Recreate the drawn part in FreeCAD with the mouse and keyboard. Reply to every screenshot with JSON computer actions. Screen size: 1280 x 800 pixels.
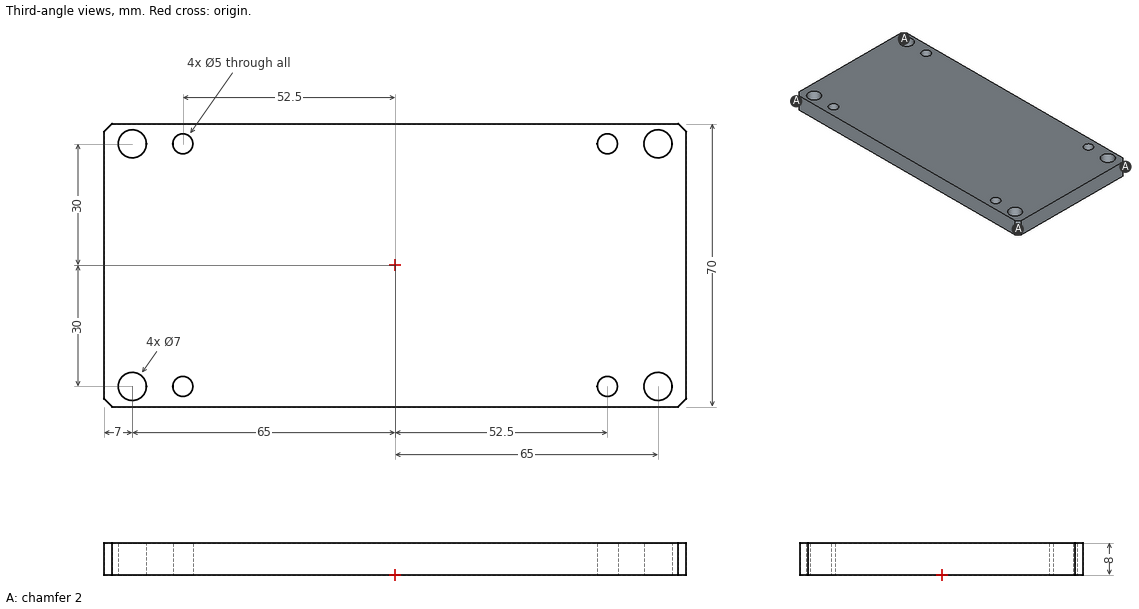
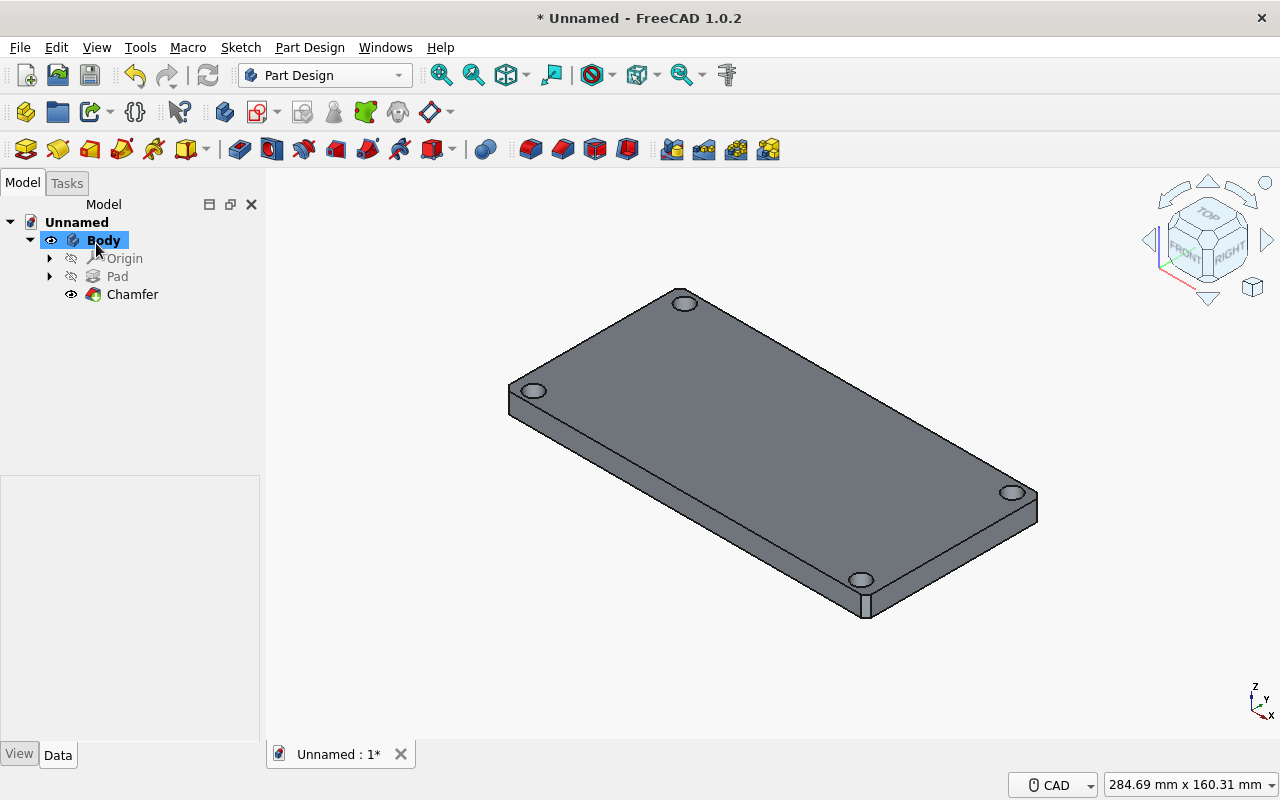
{"action": "left_click", "coordinate": [825, 471]}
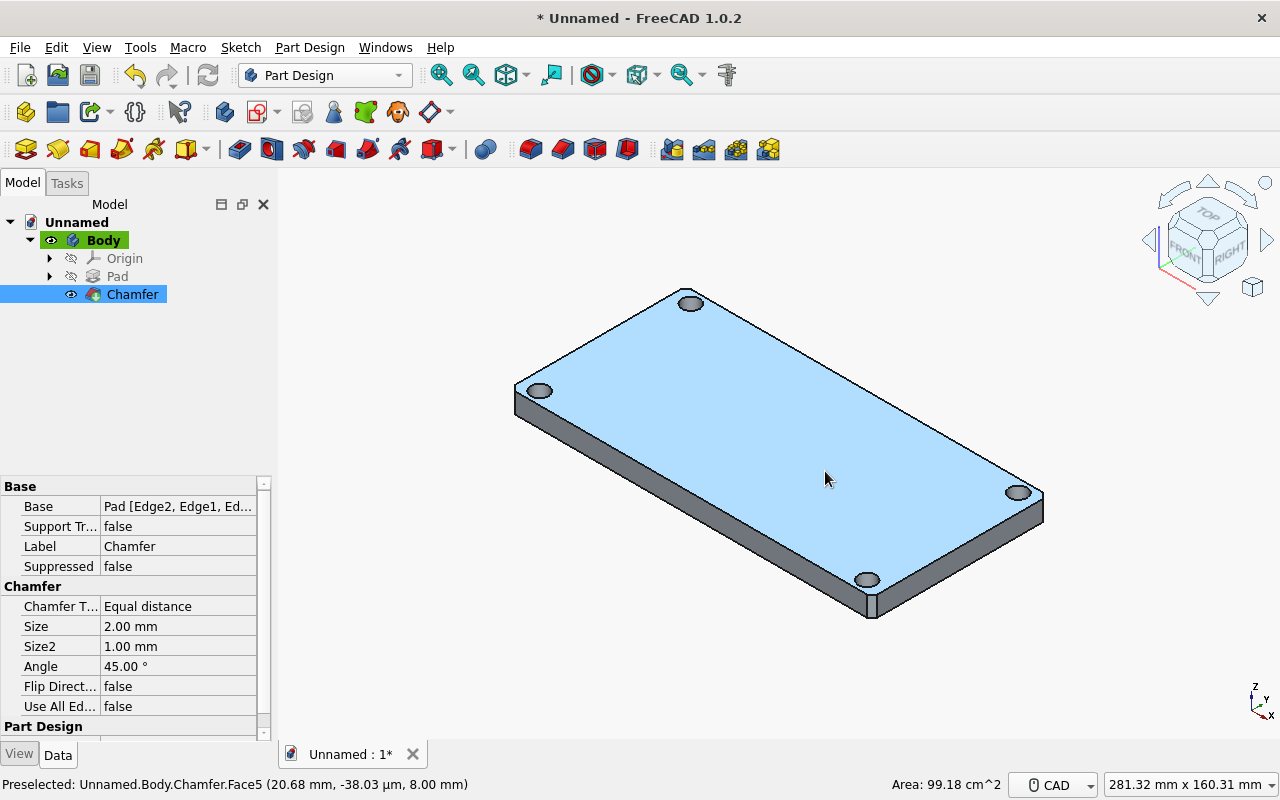
{"action": "left_click", "coordinate": [258, 112]}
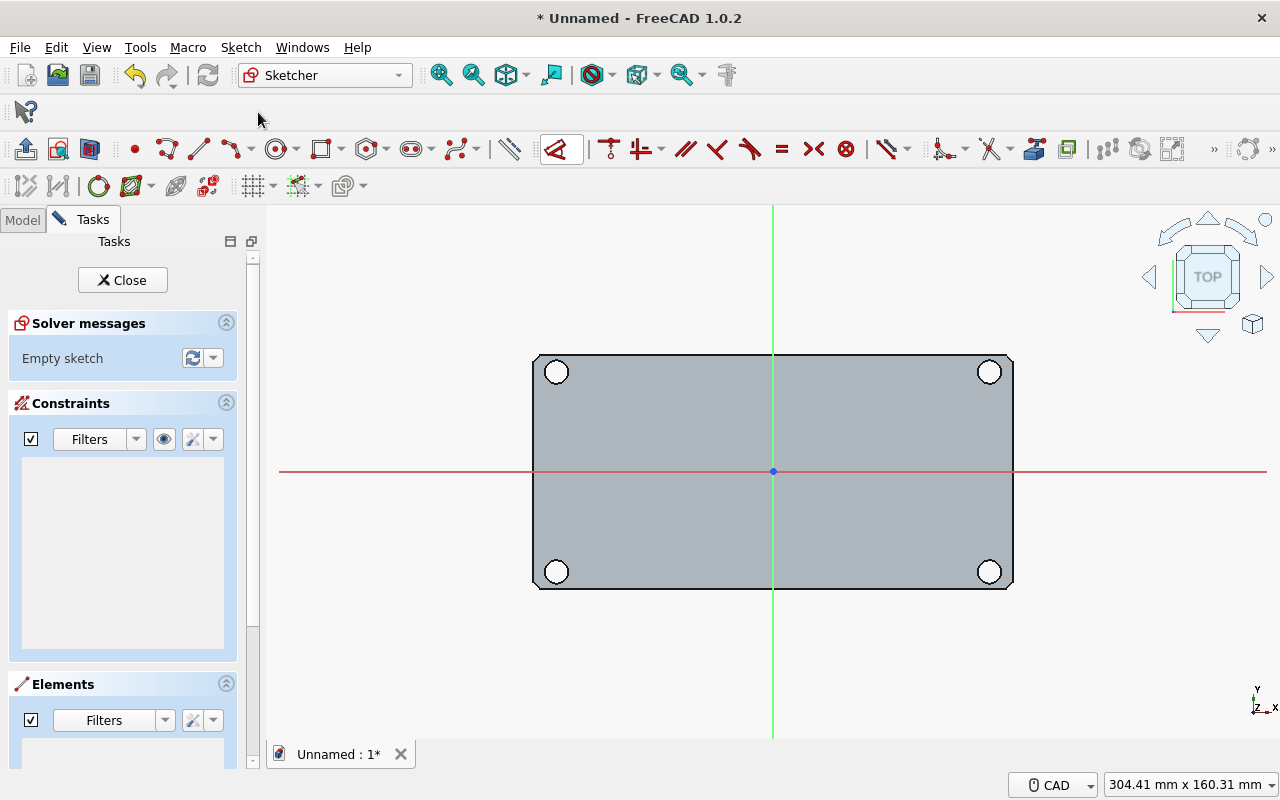
{"action": "scroll", "coordinate": [912, 472], "scroll_direction": "up", "scroll_amount": 2}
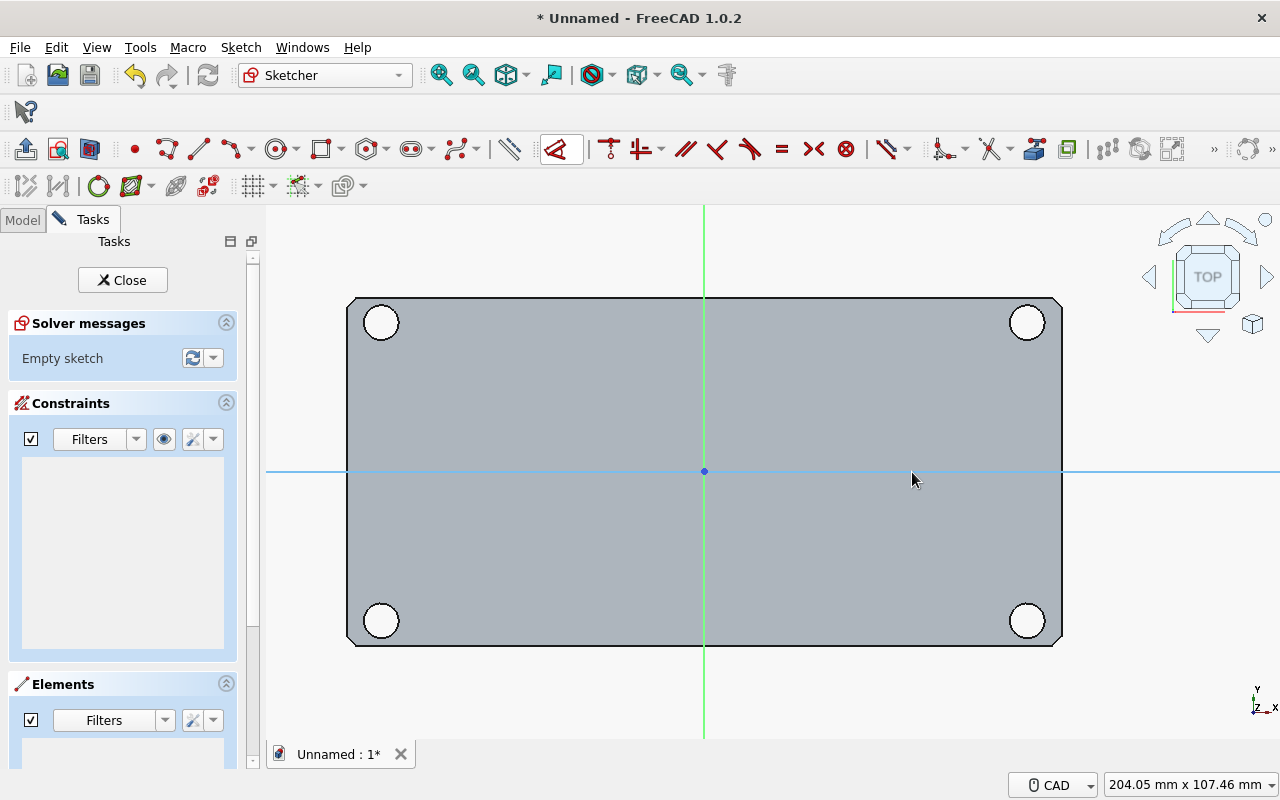
{"action": "left_click", "coordinate": [276, 150]}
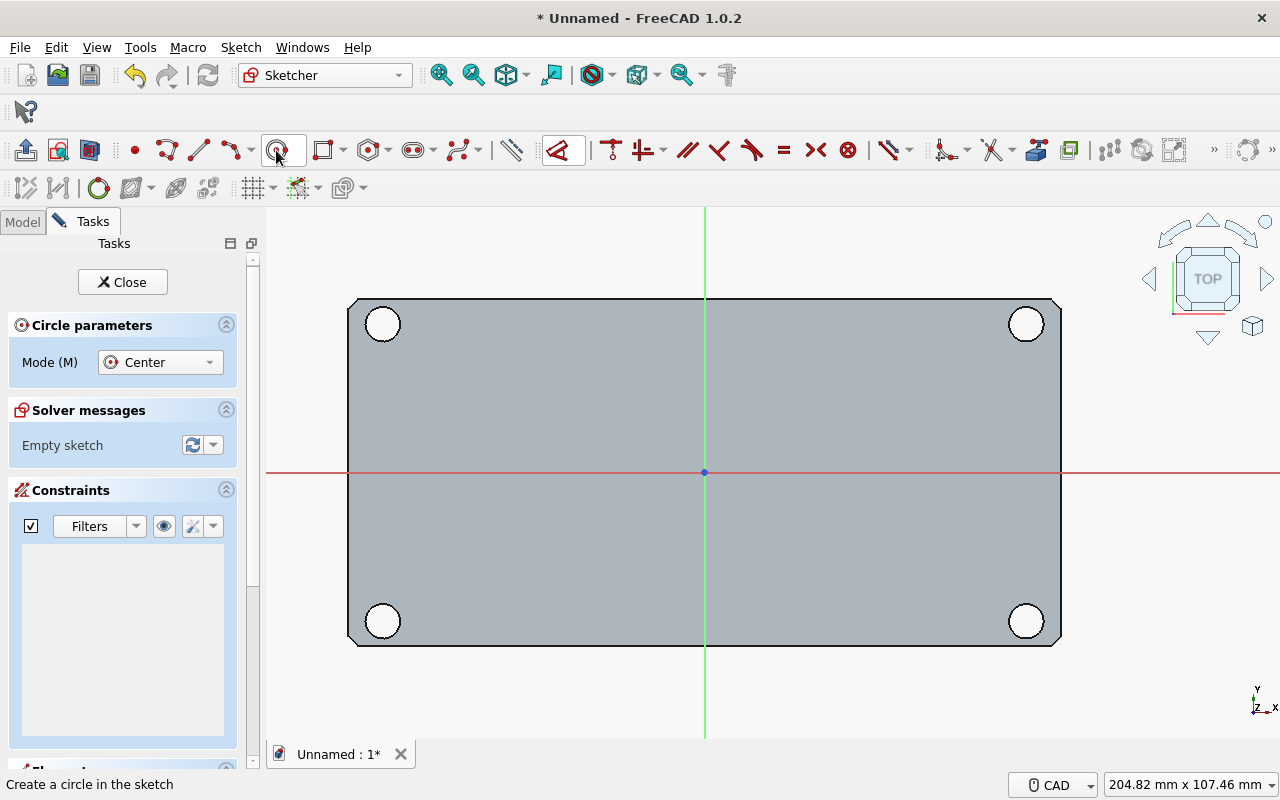
{"action": "scroll", "coordinate": [445, 324], "scroll_direction": "up", "scroll_amount": 4}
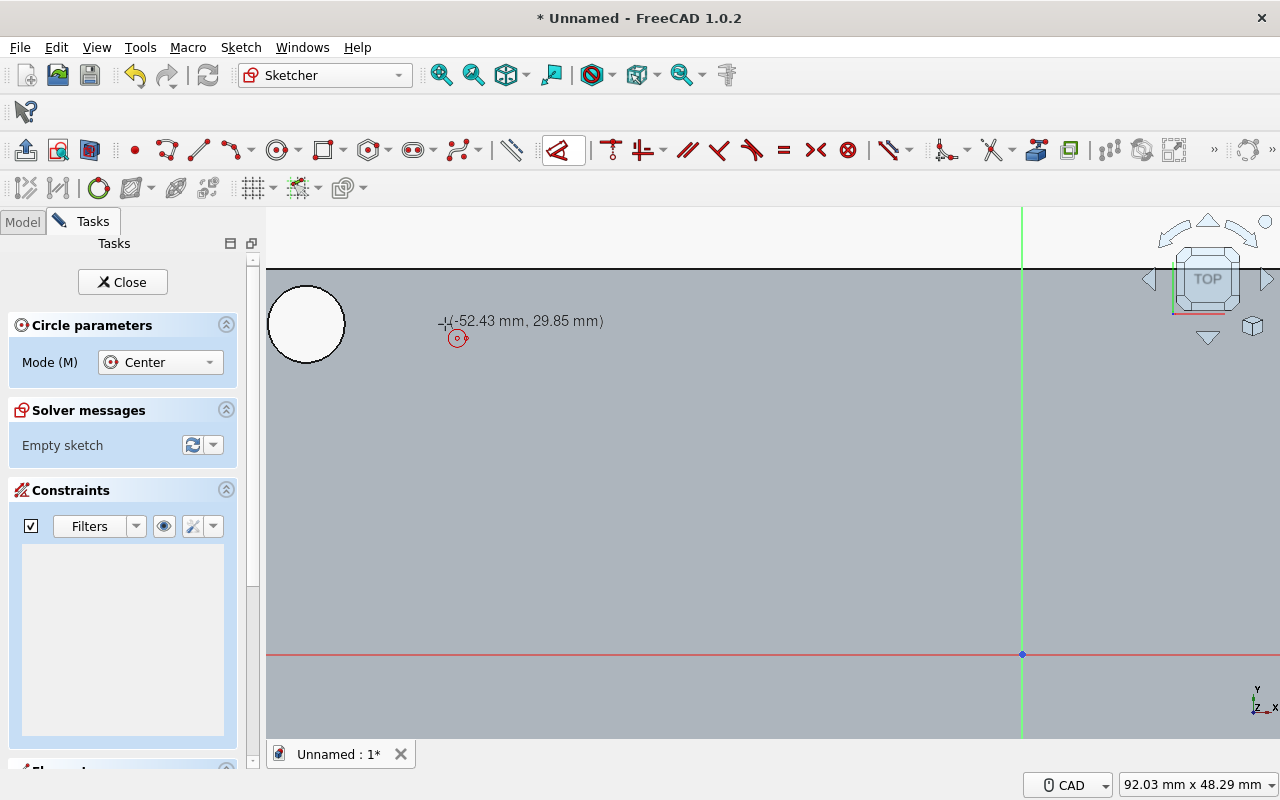
{"action": "left_click", "coordinate": [444, 324]}
{"action": "left_click", "coordinate": [464, 305]}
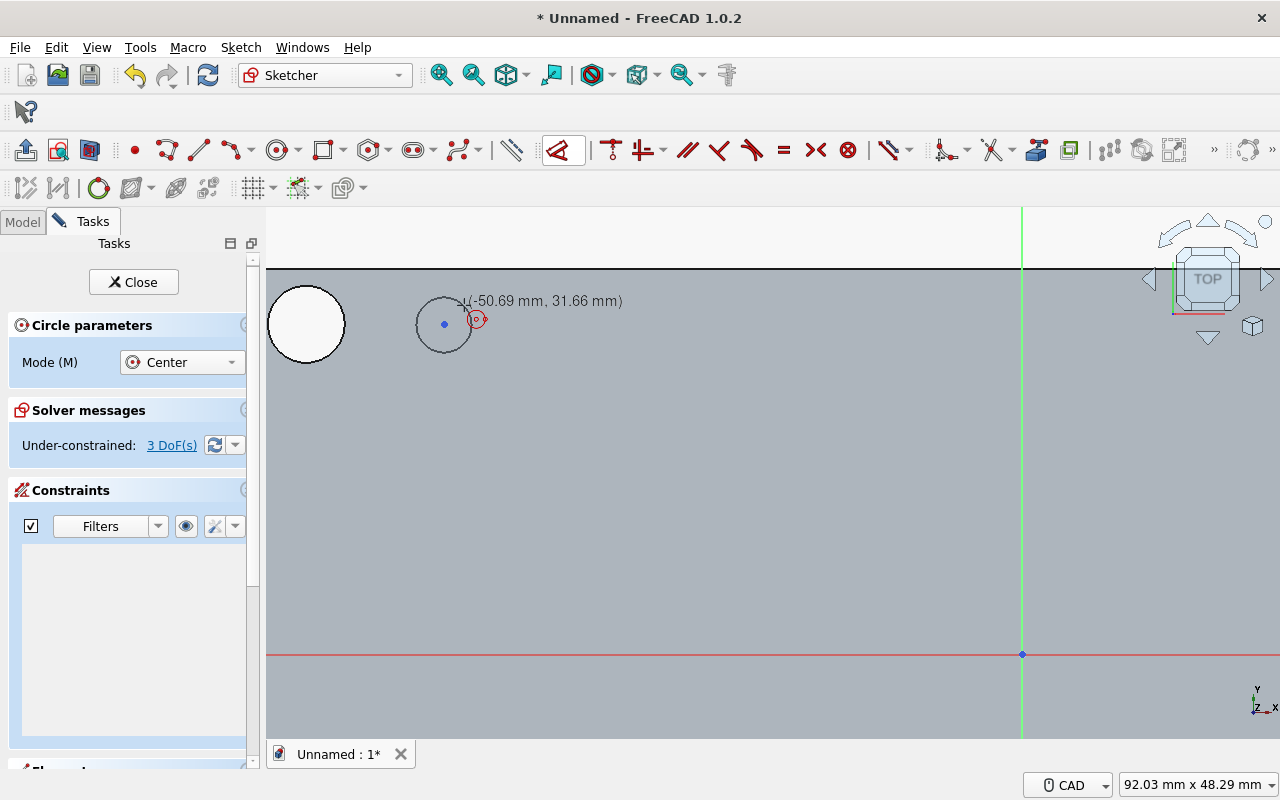
{"action": "scroll", "coordinate": [445, 325], "scroll_direction": "down", "scroll_amount": 4}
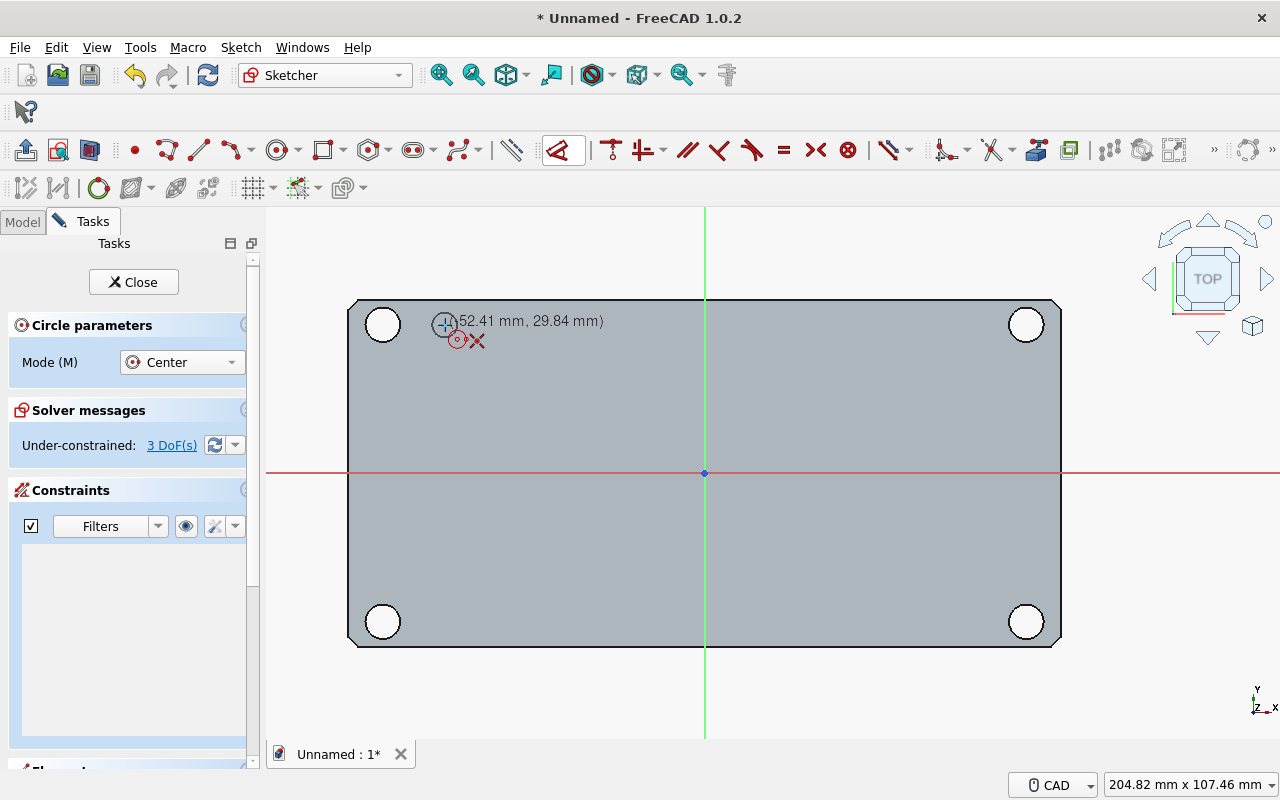
{"action": "scroll", "coordinate": [445, 622], "scroll_direction": "up", "scroll_amount": 4}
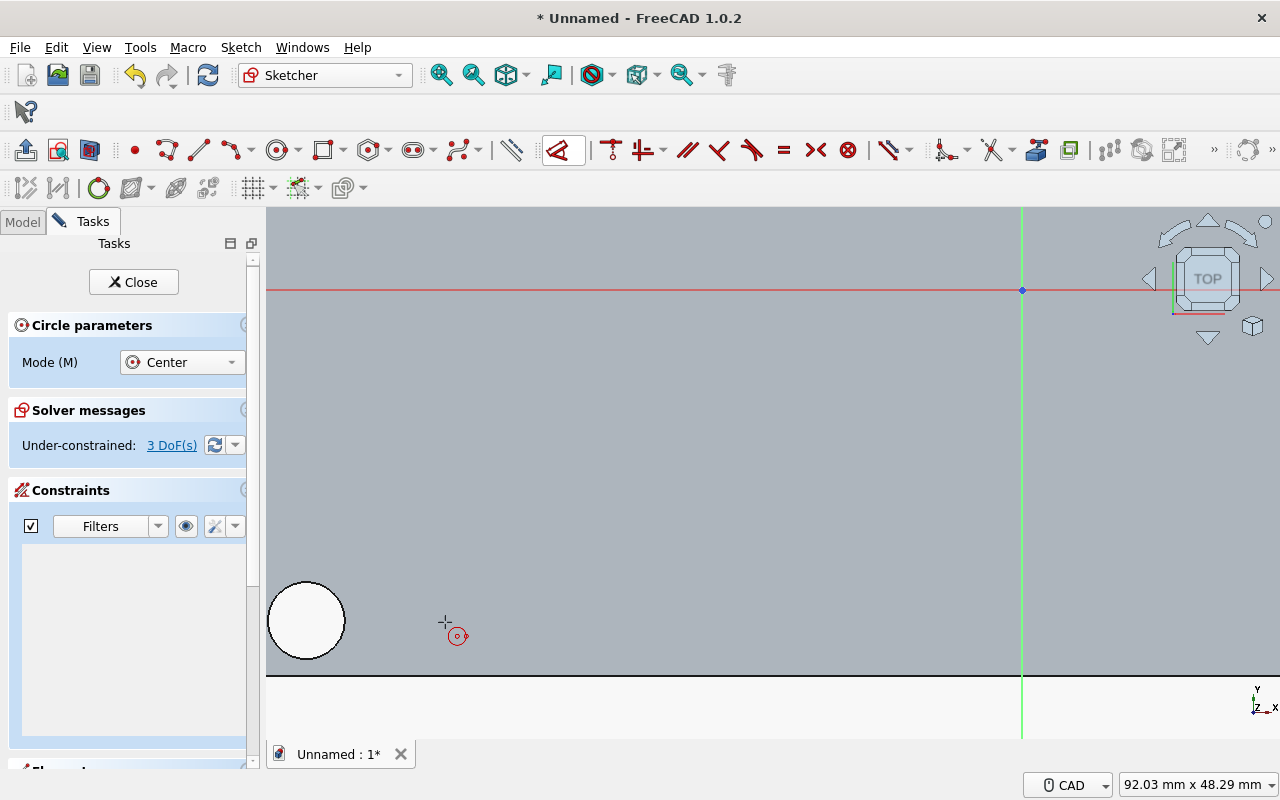
{"action": "left_click", "coordinate": [444, 621]}
{"action": "left_click", "coordinate": [464, 601]}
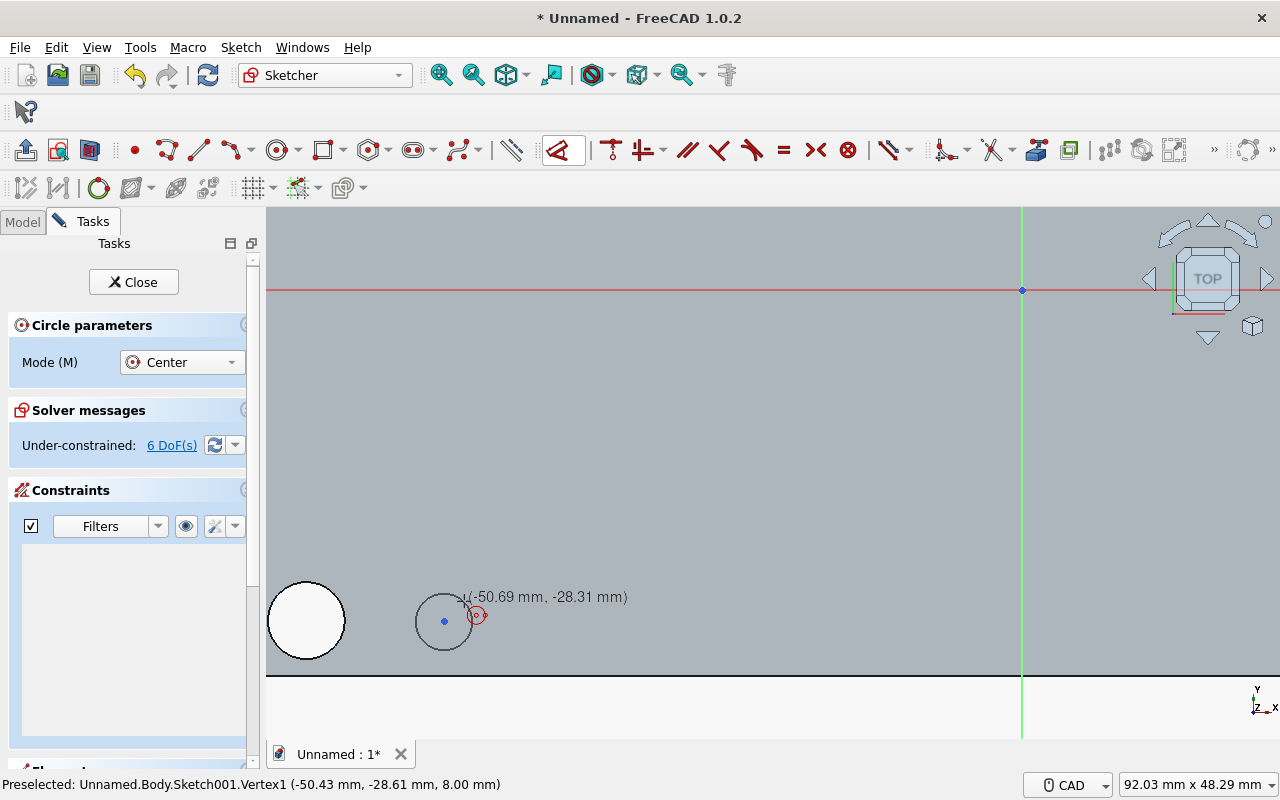
{"action": "scroll", "coordinate": [445, 622], "scroll_direction": "down", "scroll_amount": 4}